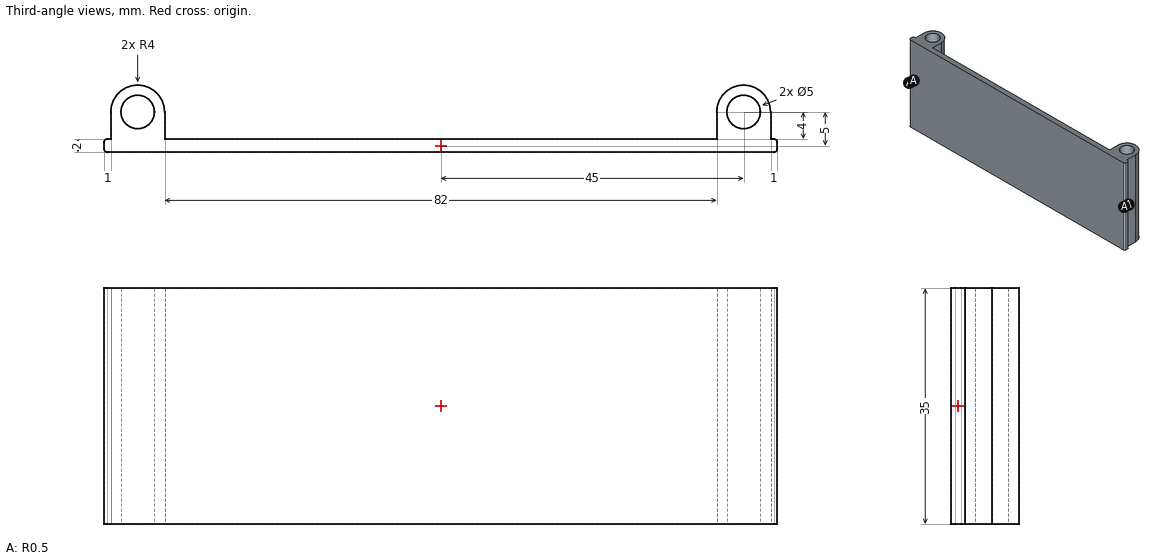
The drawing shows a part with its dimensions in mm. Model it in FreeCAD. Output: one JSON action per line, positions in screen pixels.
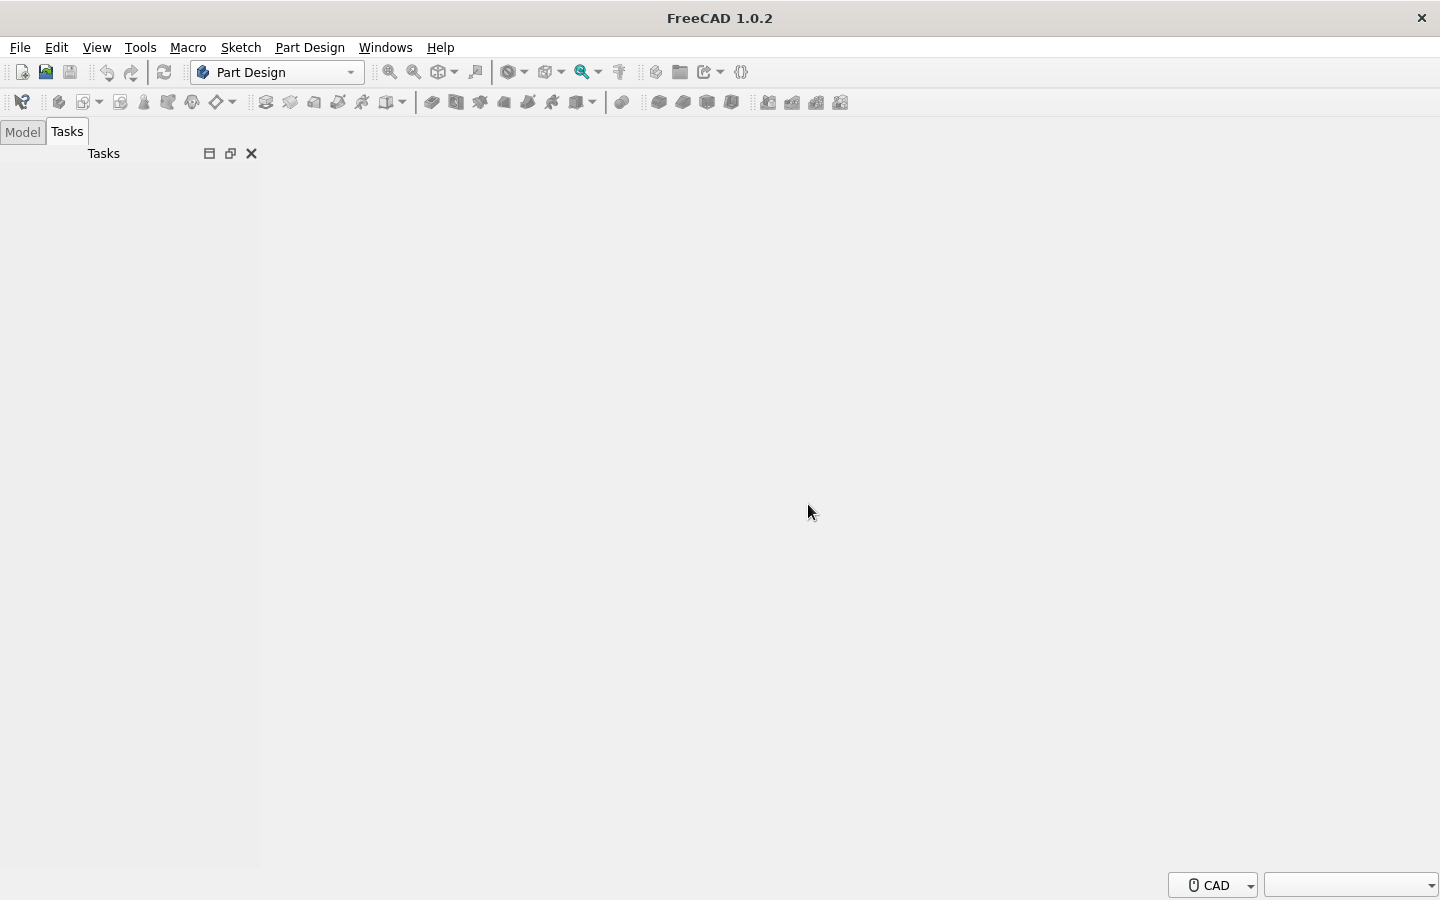
{"action": "left_click", "coordinate": [22, 72]}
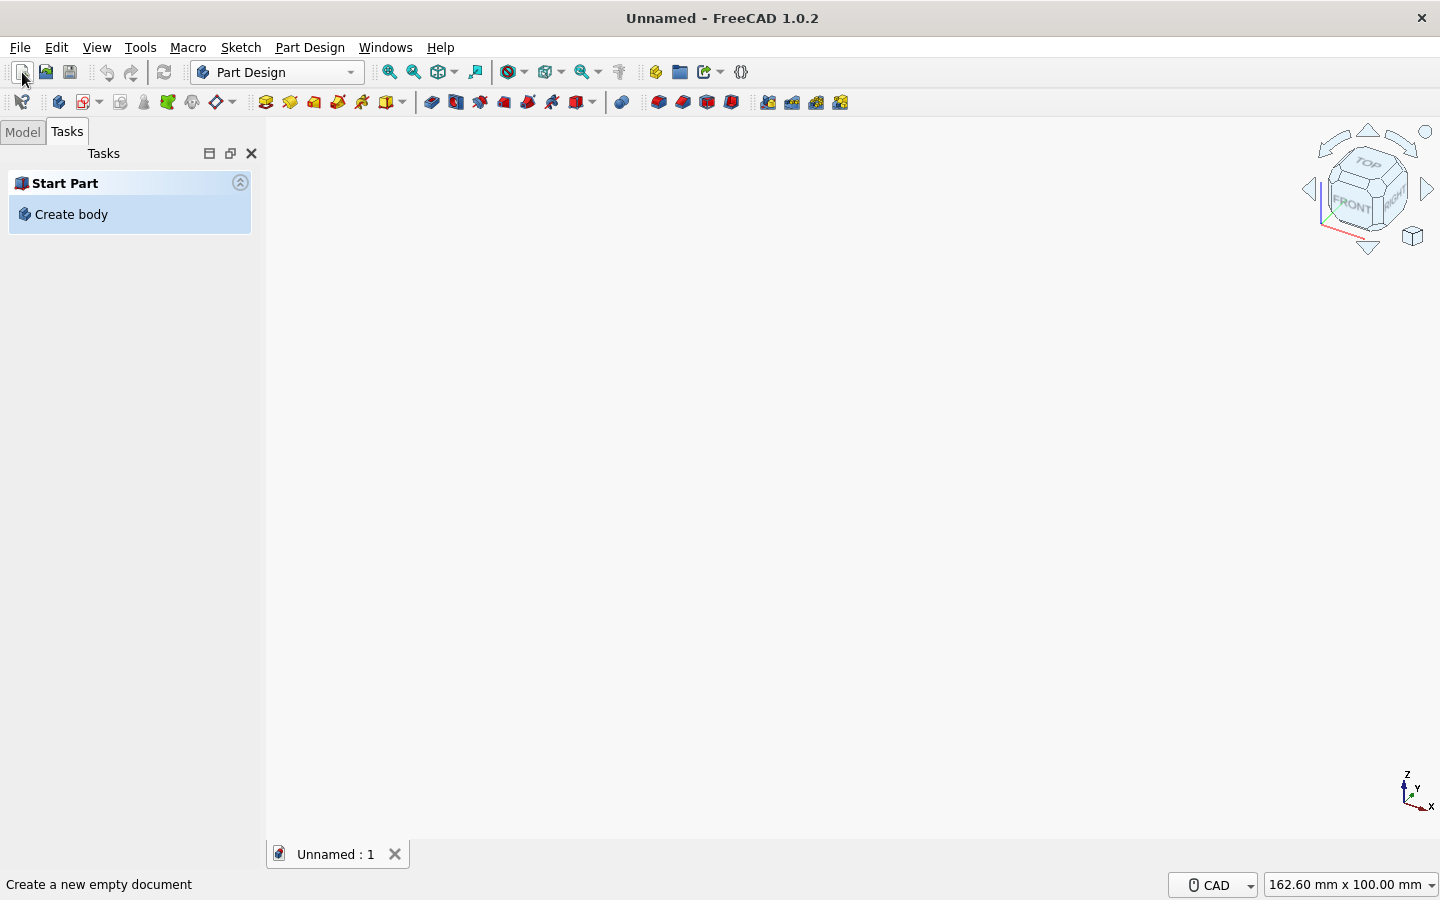
{"action": "left_click", "coordinate": [84, 102]}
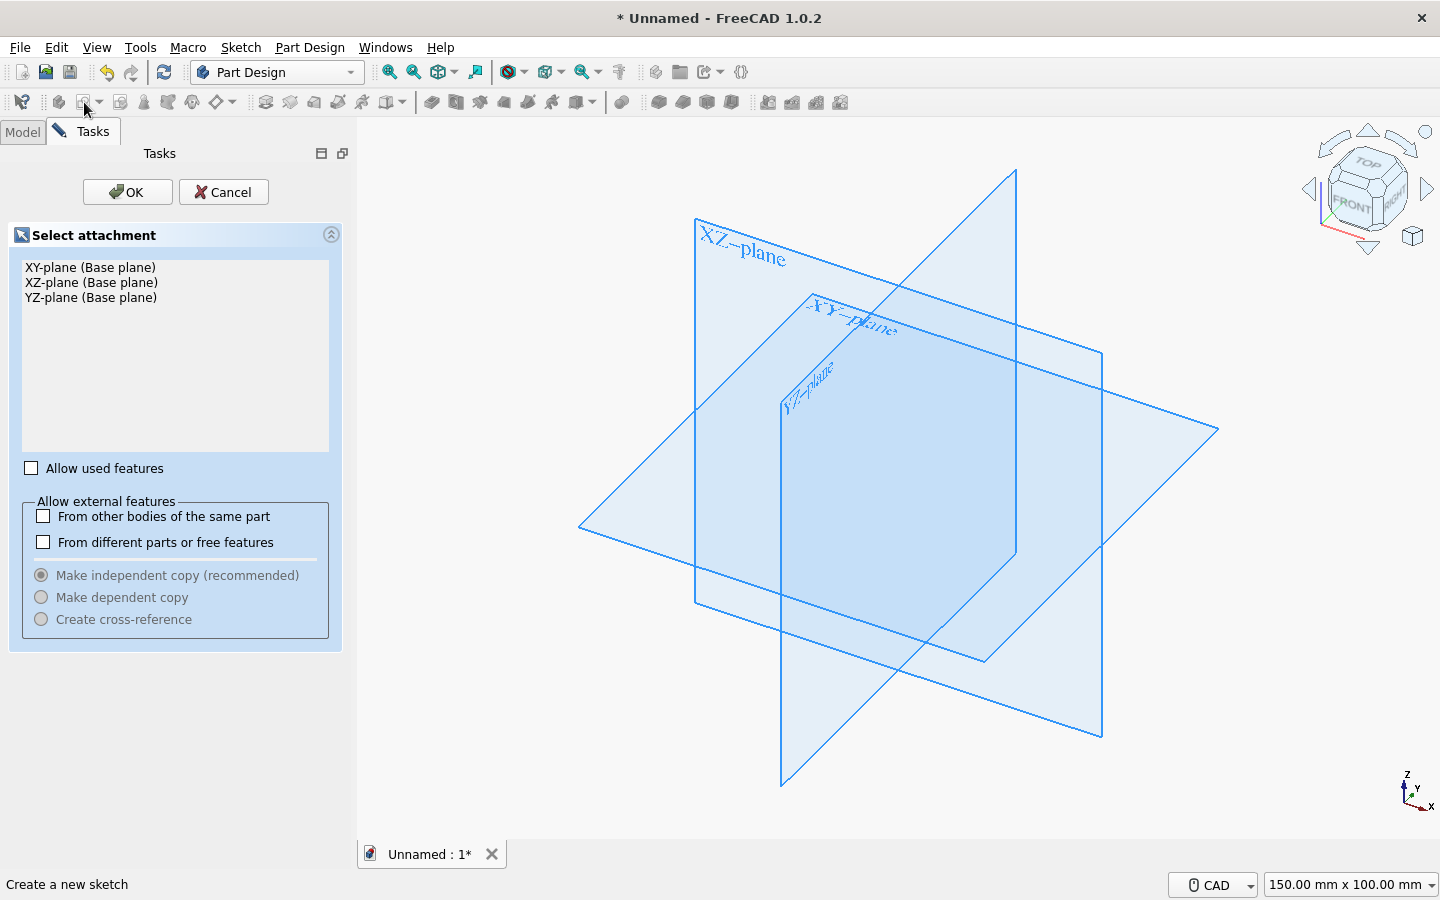
{"action": "left_click", "coordinate": [82, 268]}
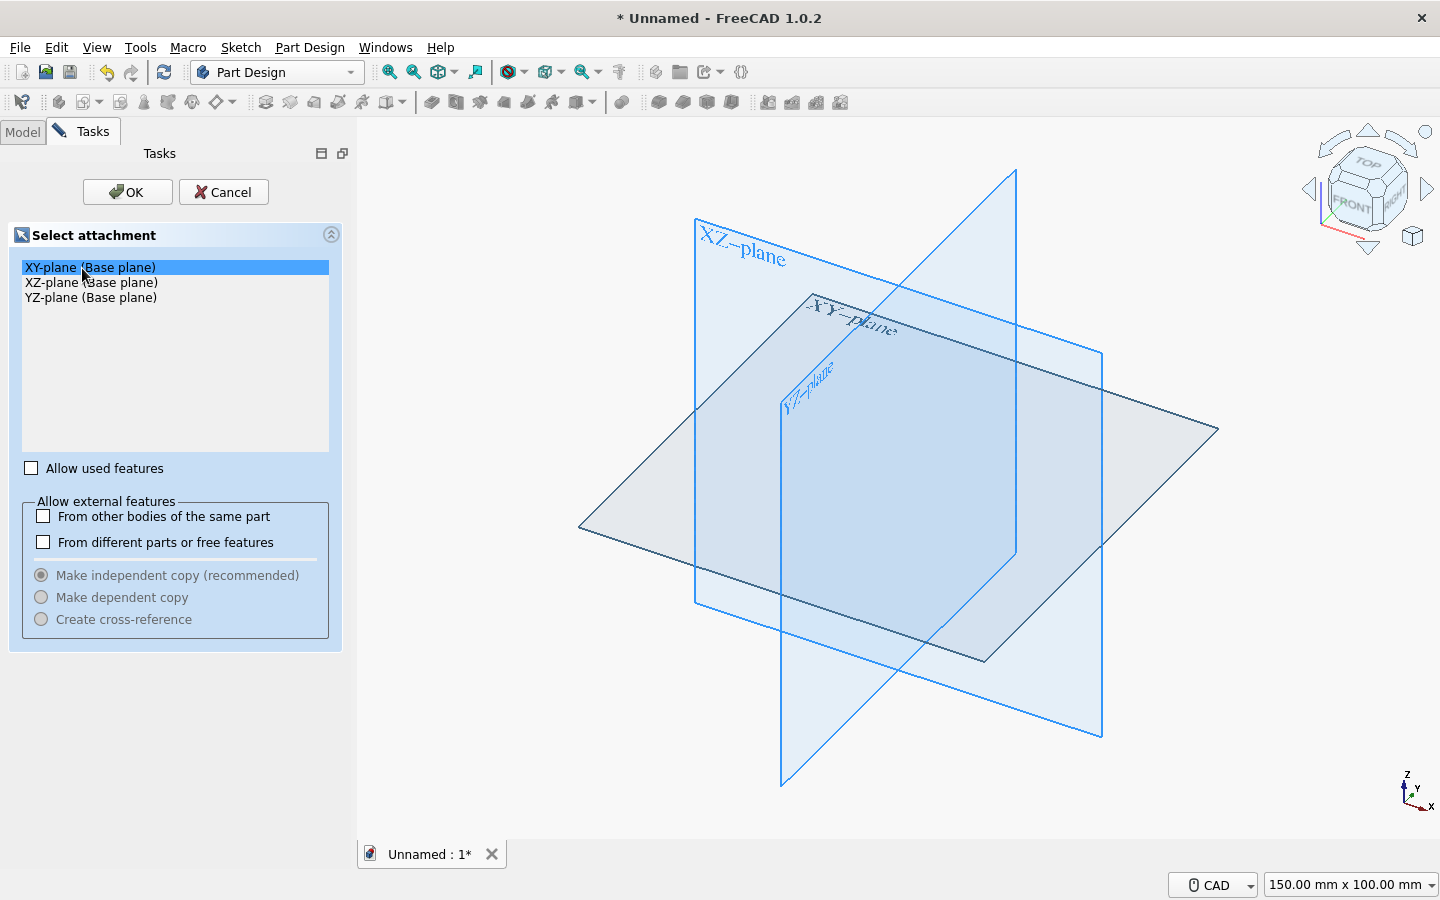
{"action": "left_click", "coordinate": [128, 192]}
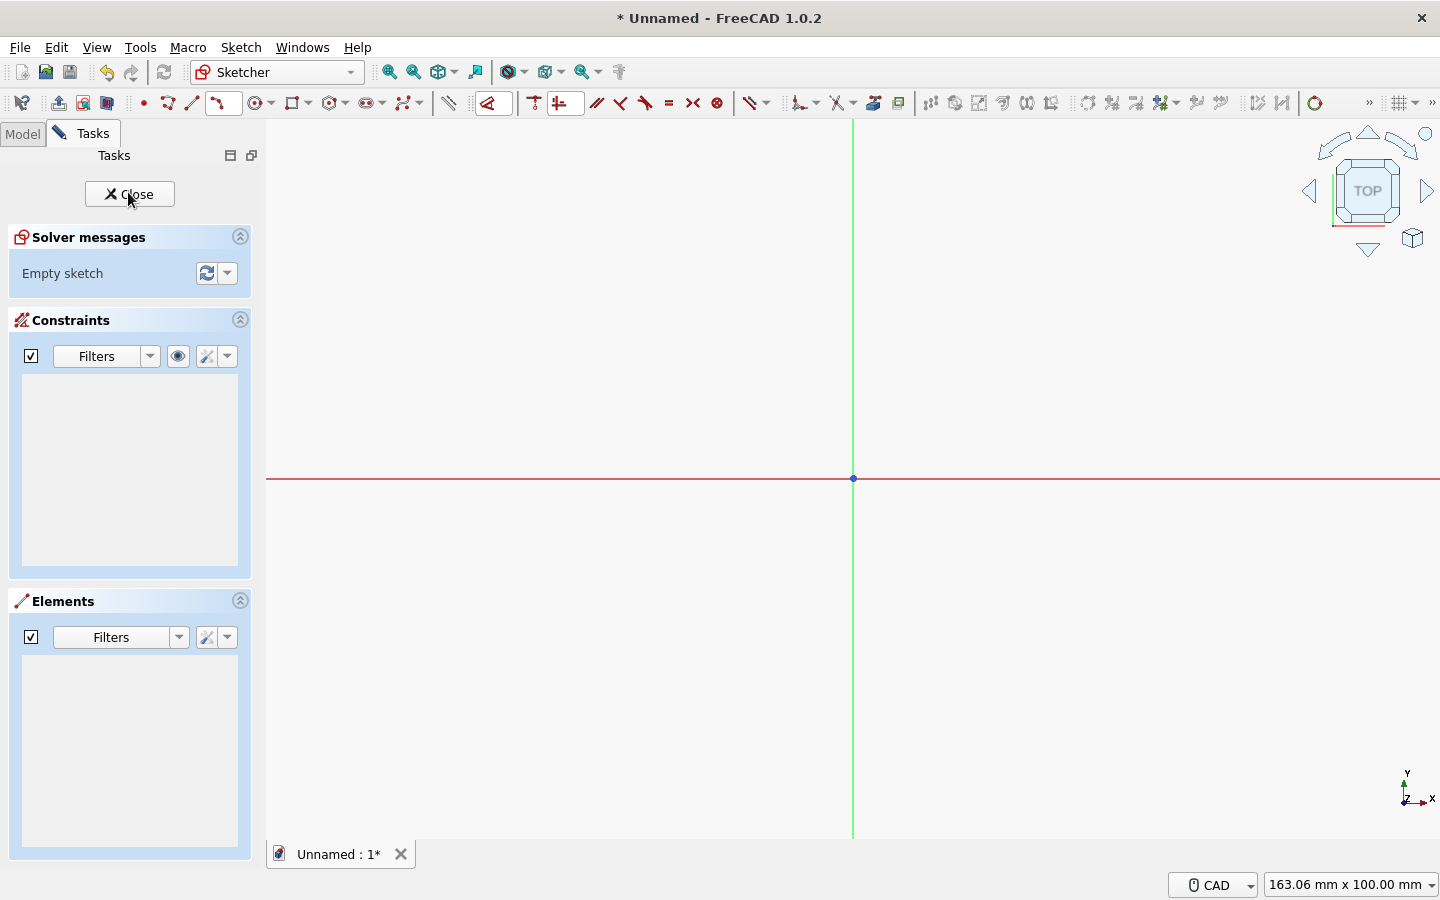
{"action": "left_click", "coordinate": [168, 104]}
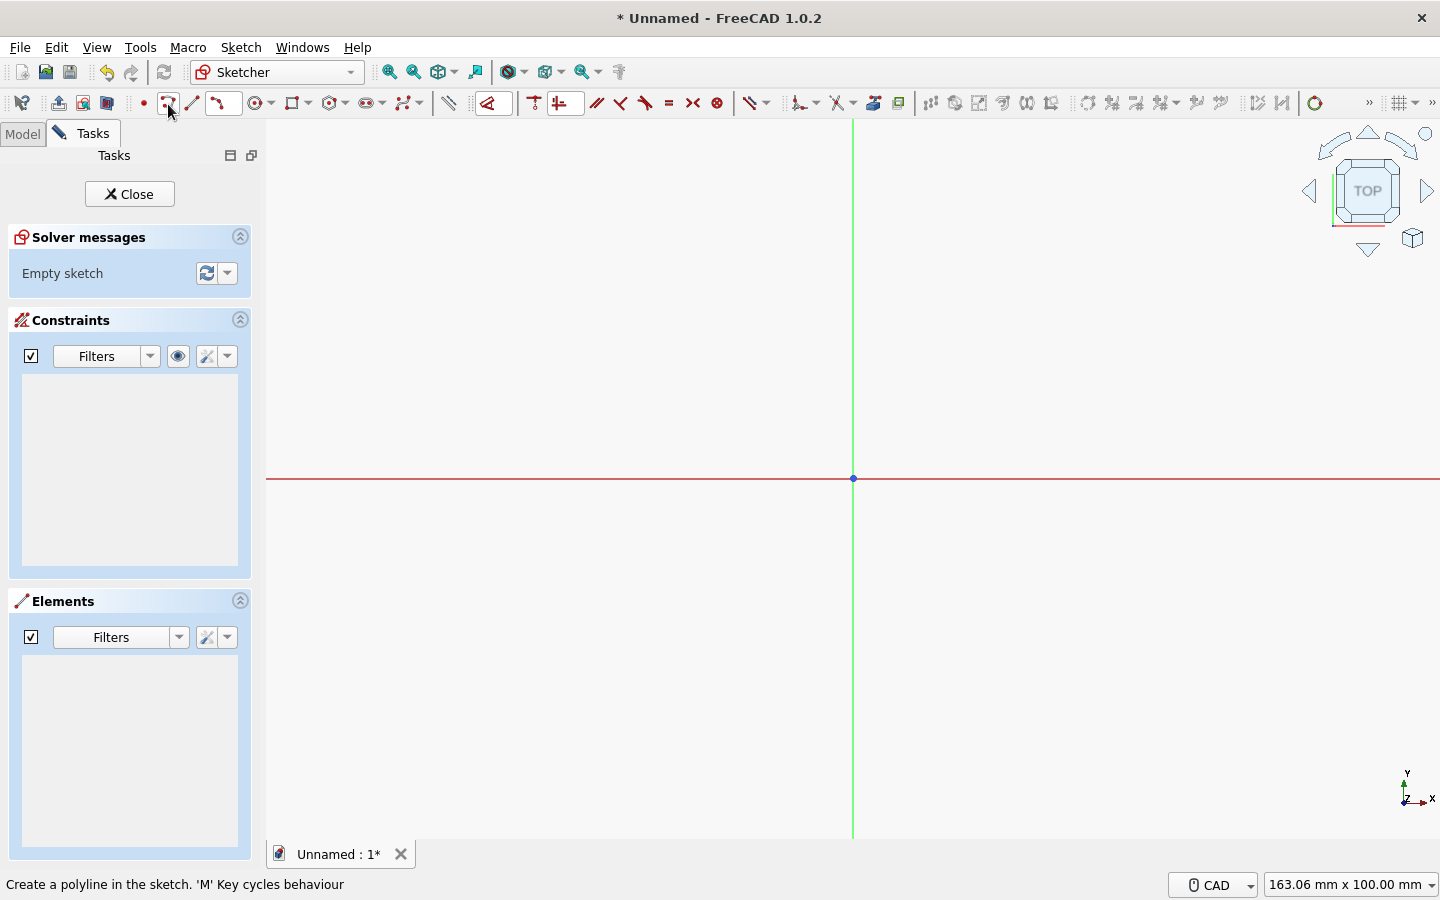
{"action": "left_click", "coordinate": [1148, 443]}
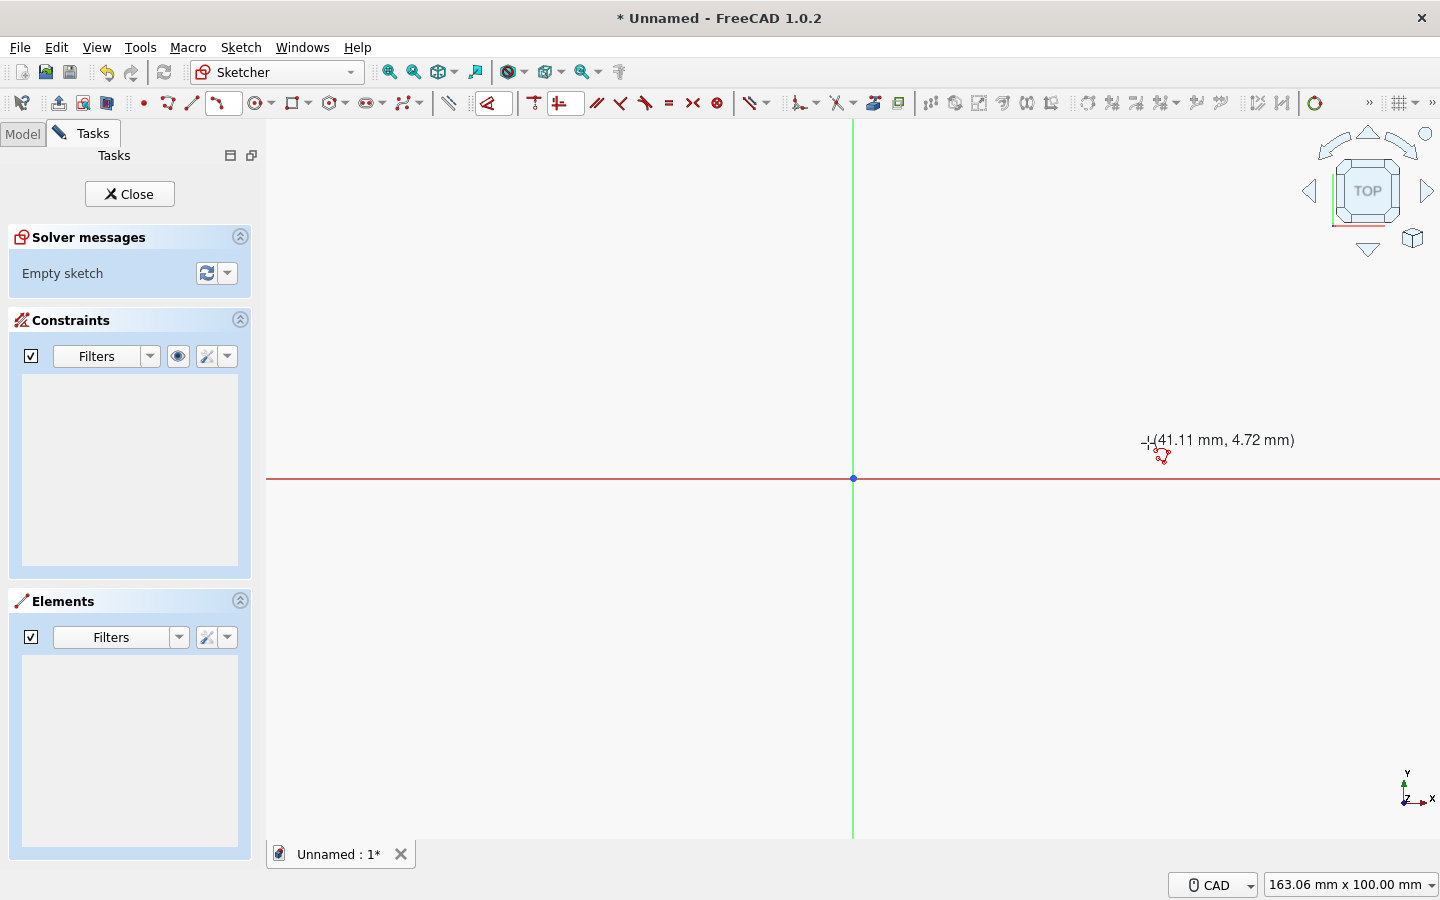
{"action": "scroll", "coordinate": [1148, 472], "scroll_direction": "up", "scroll_amount": 4}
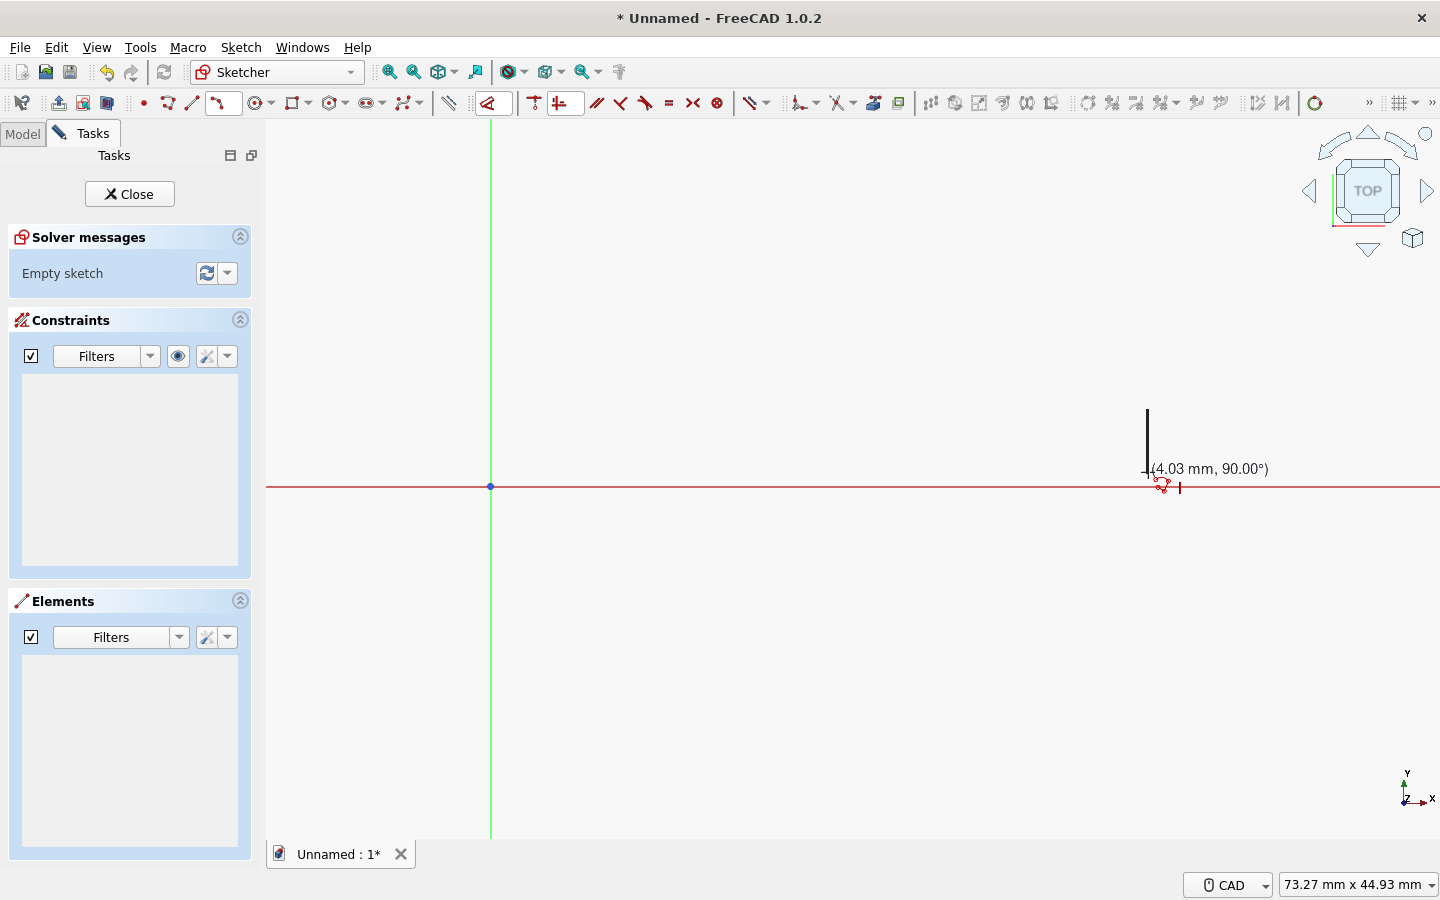
{"action": "left_click", "coordinate": [1147, 471]}